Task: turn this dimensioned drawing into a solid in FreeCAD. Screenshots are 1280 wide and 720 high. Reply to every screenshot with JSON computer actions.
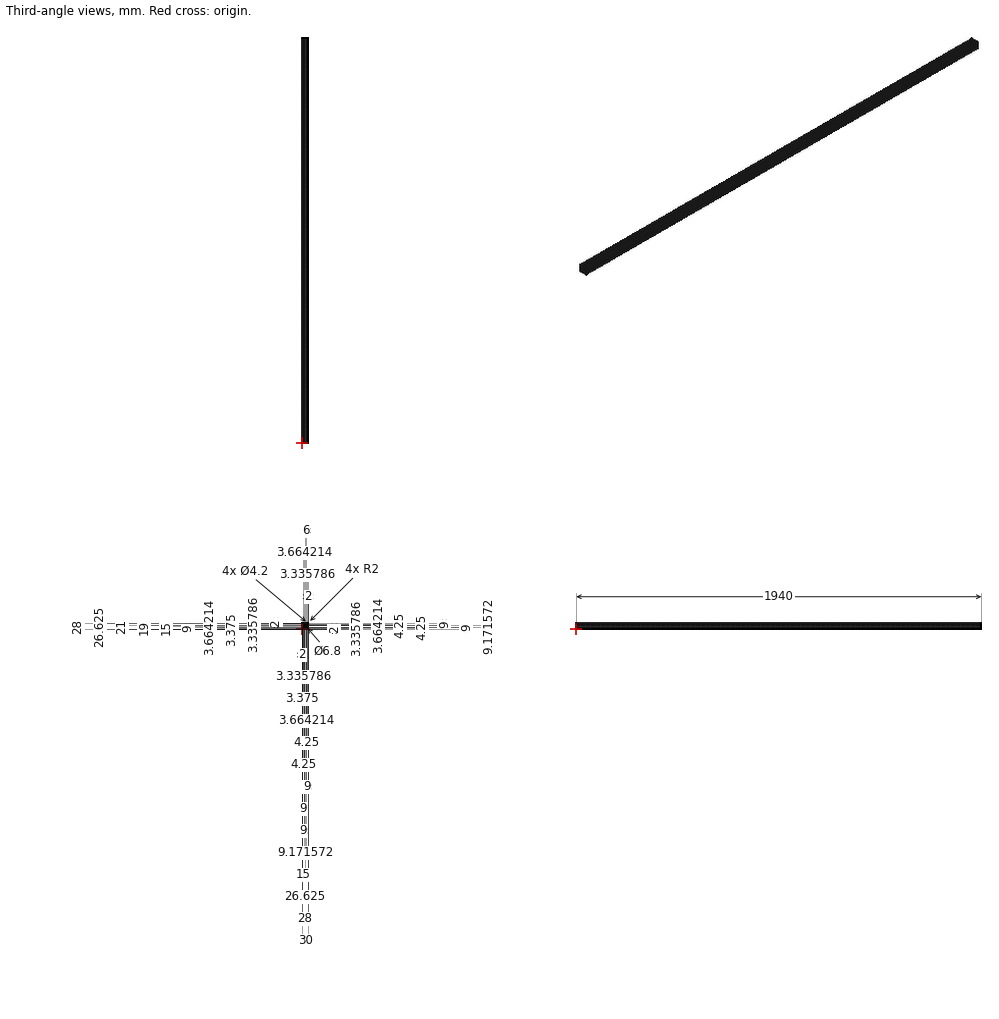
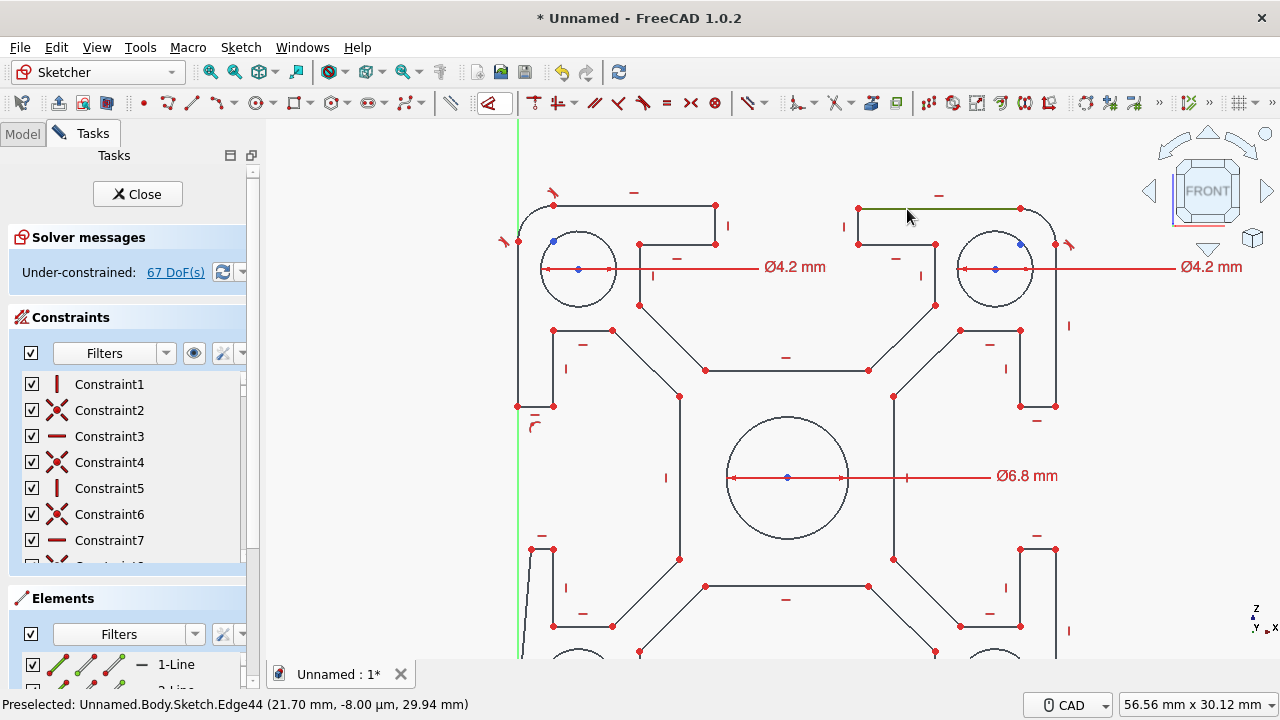
{"action": "left_click", "coordinate": [1052, 228]}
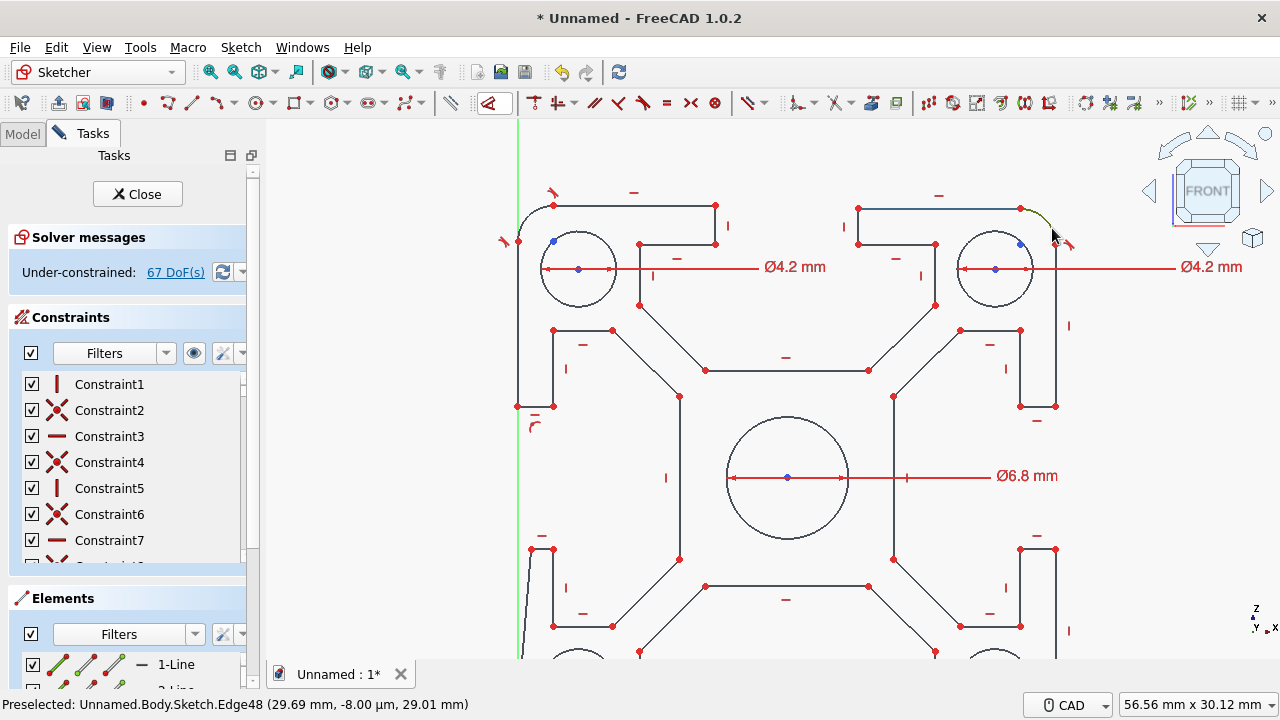
{"action": "left_click", "coordinate": [644, 104]}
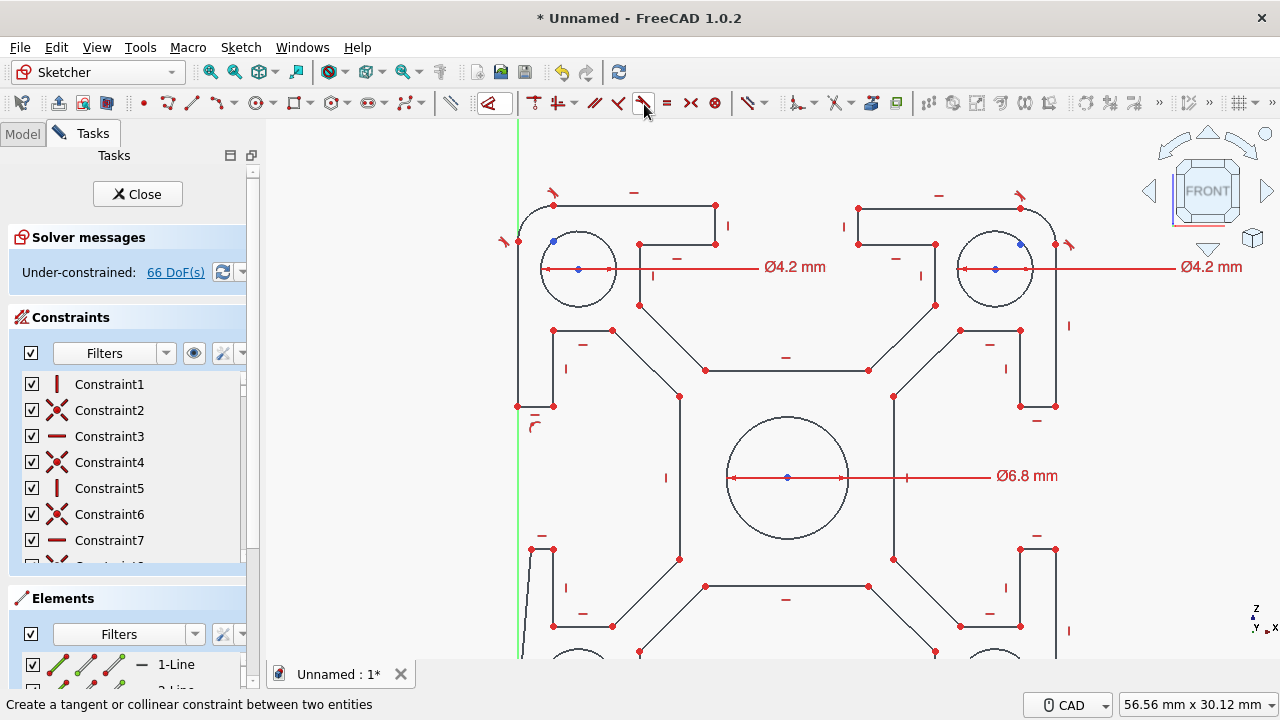
{"action": "scroll", "coordinate": [537, 211], "scroll_direction": "down", "scroll_amount": 2}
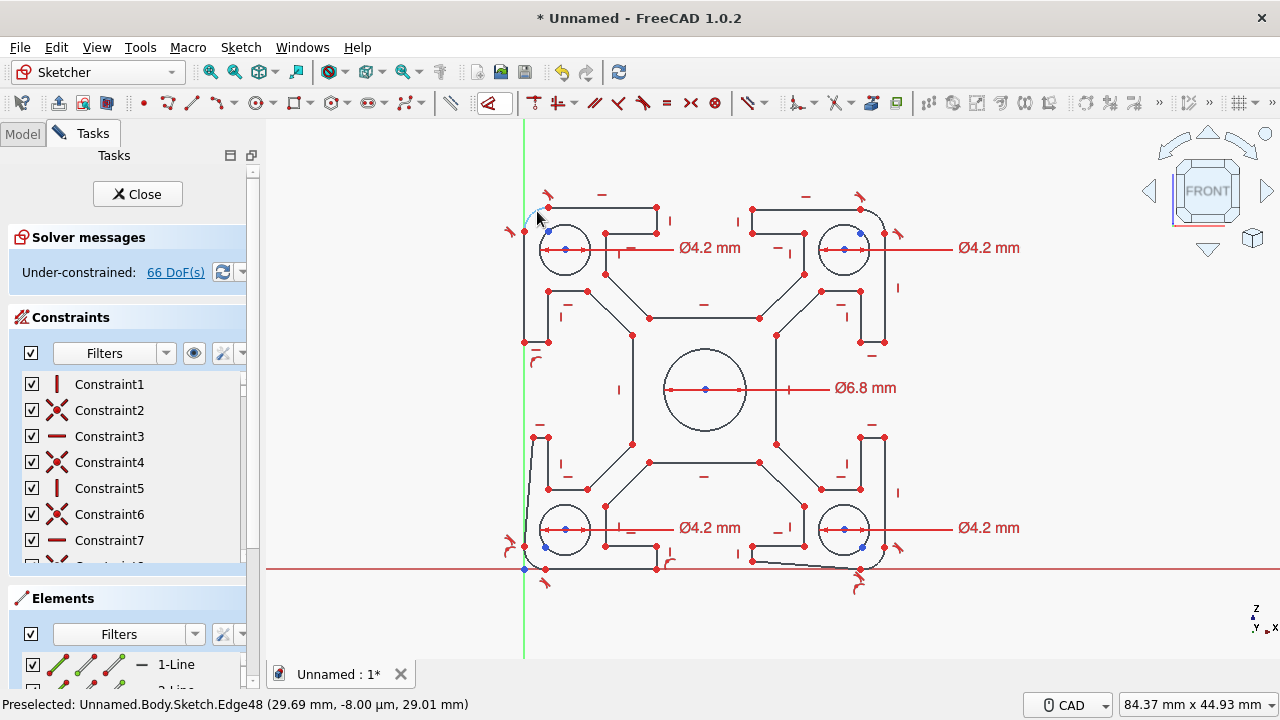
{"action": "left_click", "coordinate": [828, 567]}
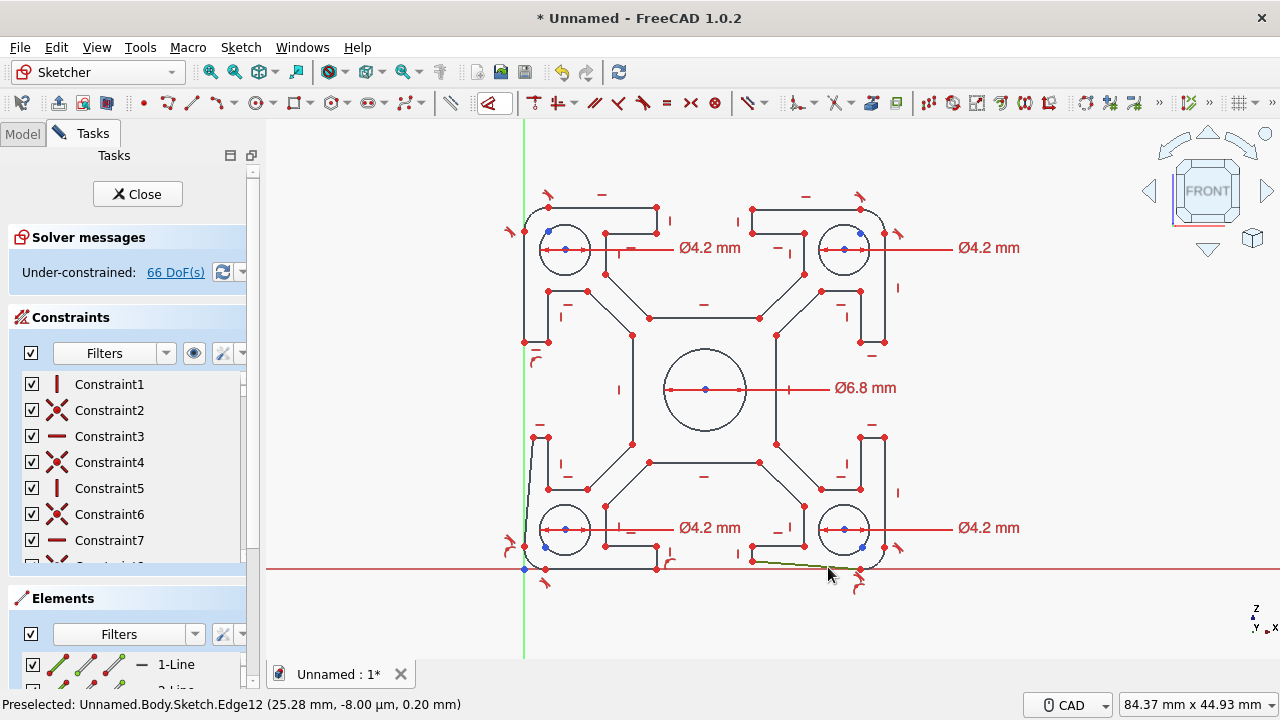
{"action": "left_click", "coordinate": [576, 104]}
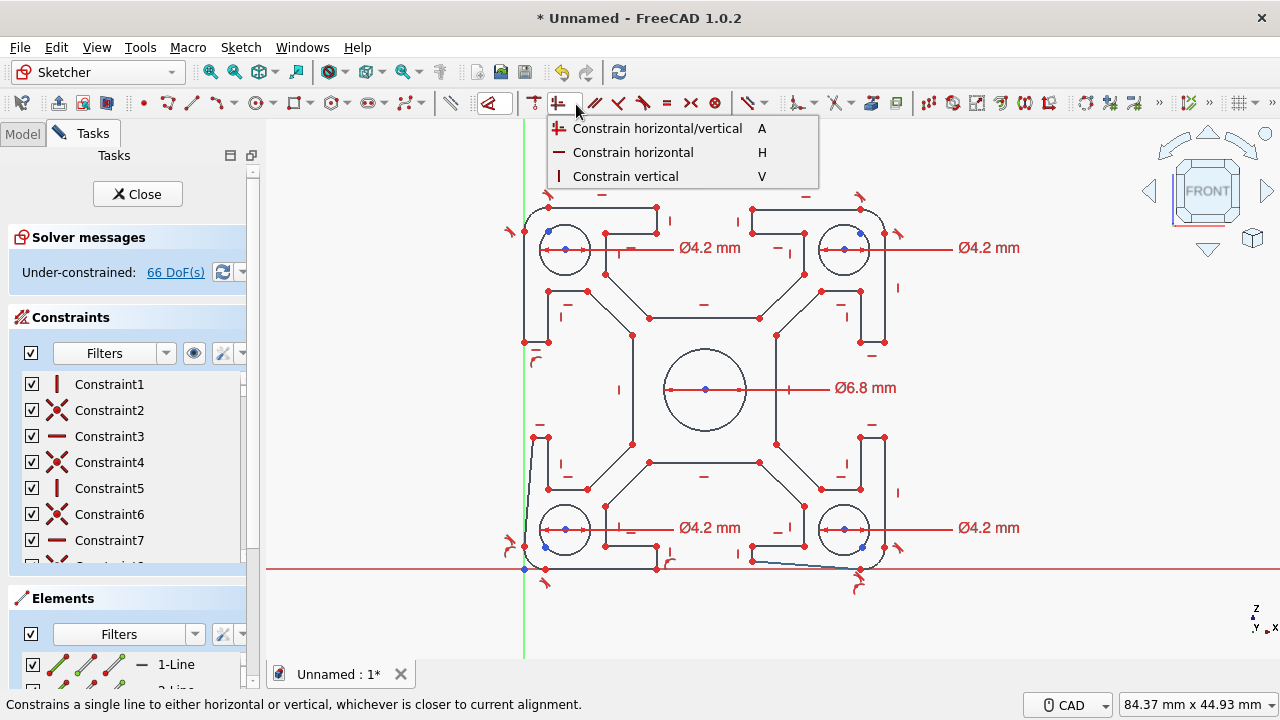
{"action": "left_click", "coordinate": [683, 152]}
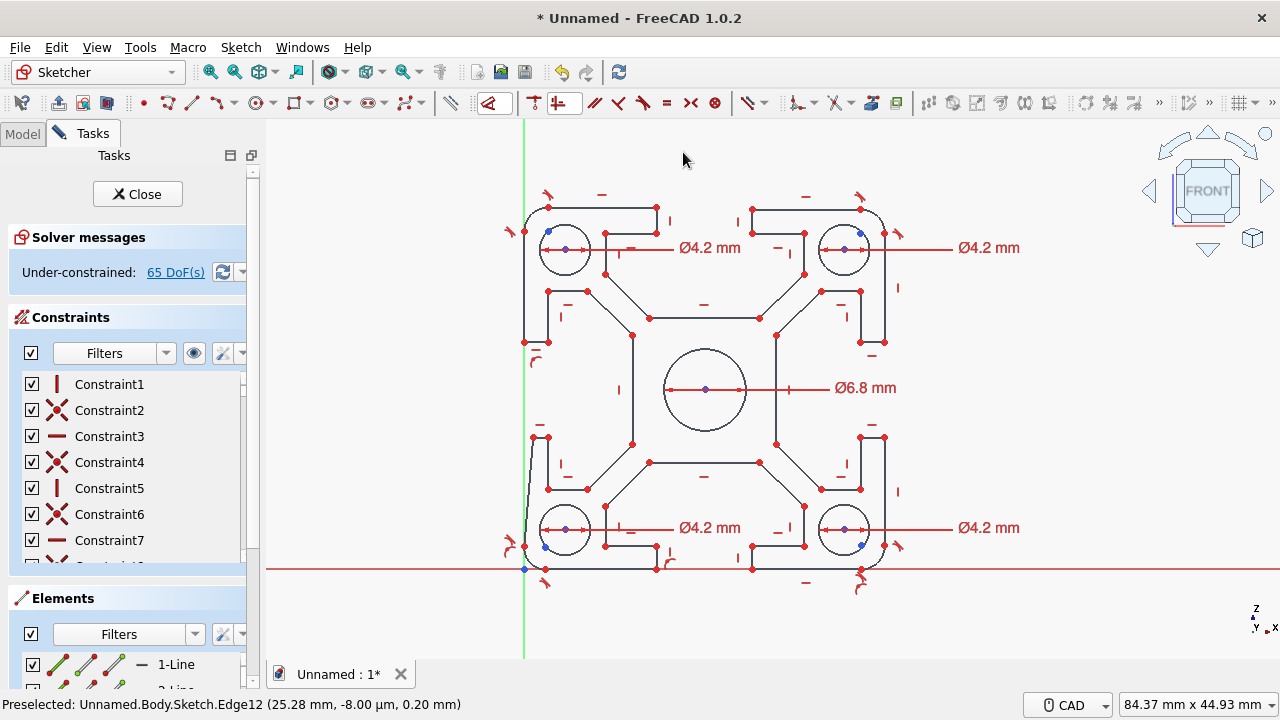
{"action": "left_click", "coordinate": [623, 569]}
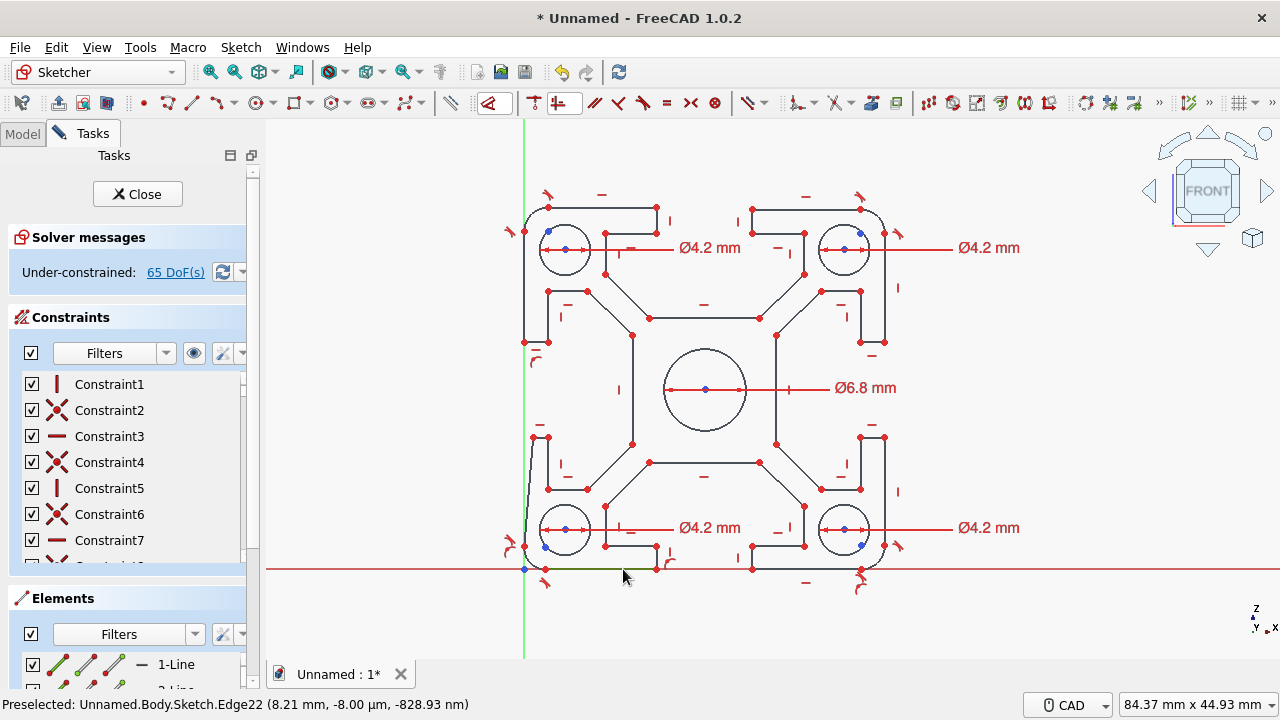
{"action": "key", "text": "h"}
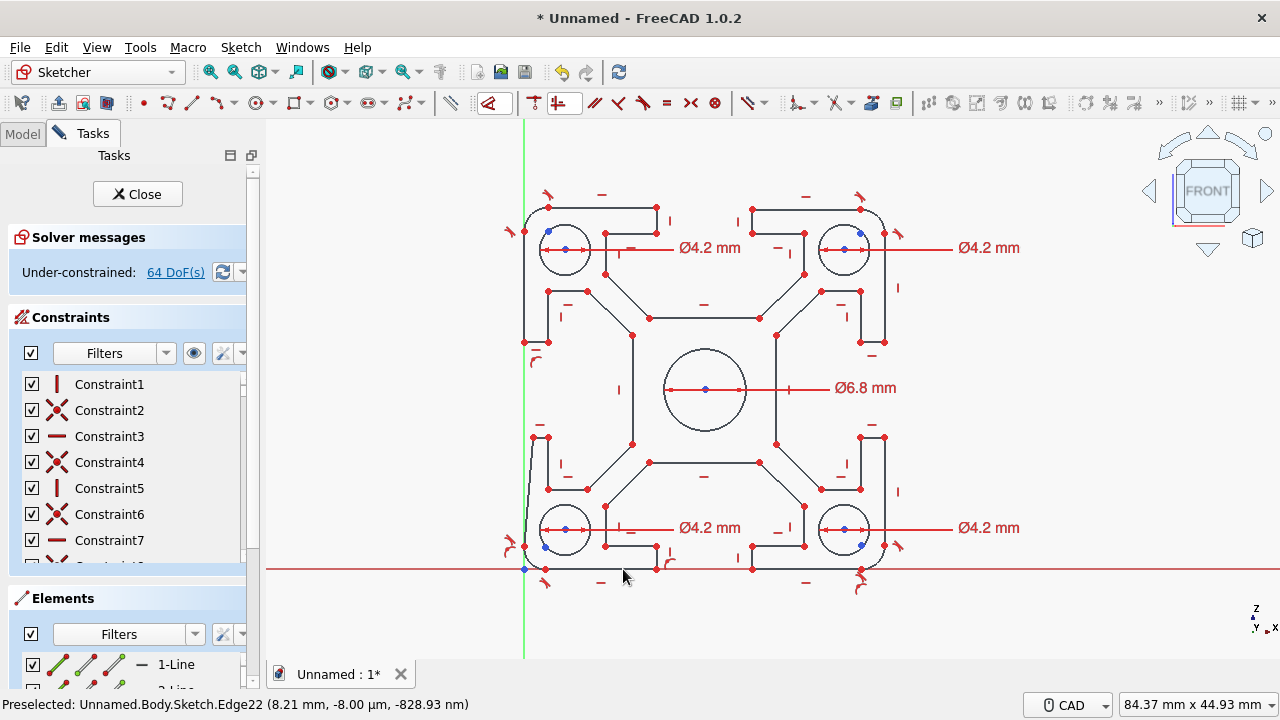
{"action": "left_click", "coordinate": [527, 514]}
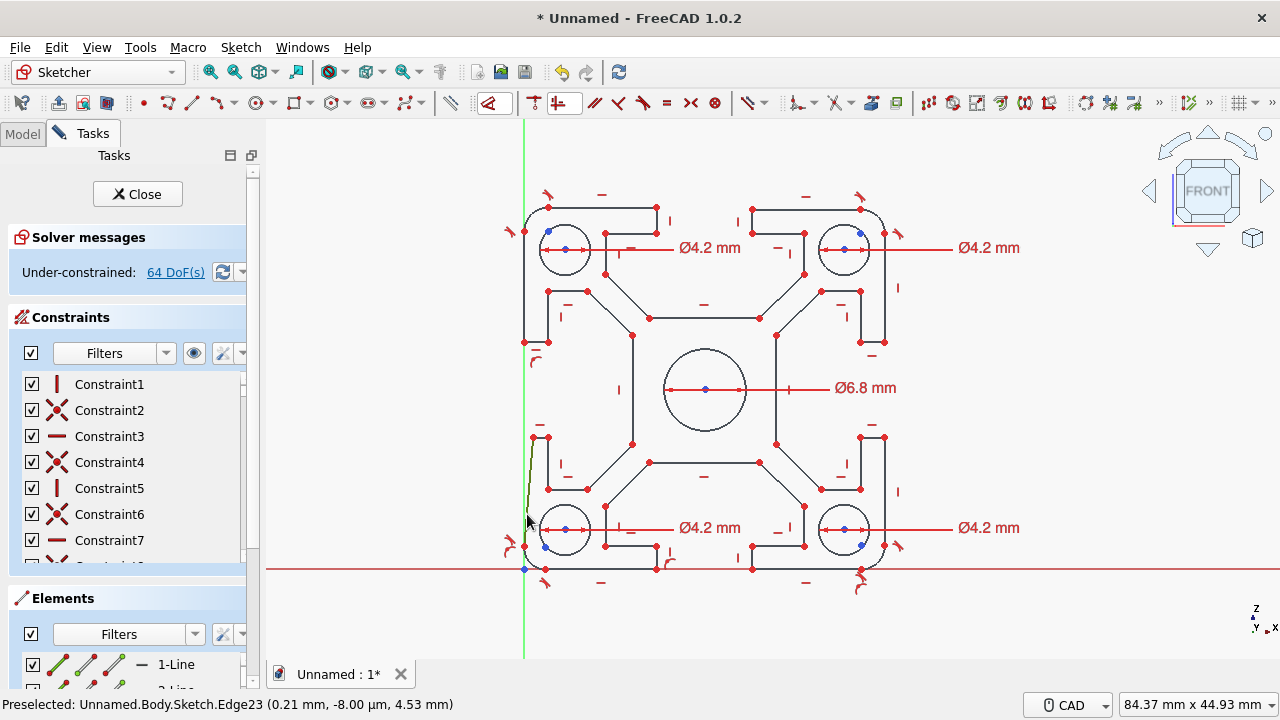
{"action": "key", "text": "v"}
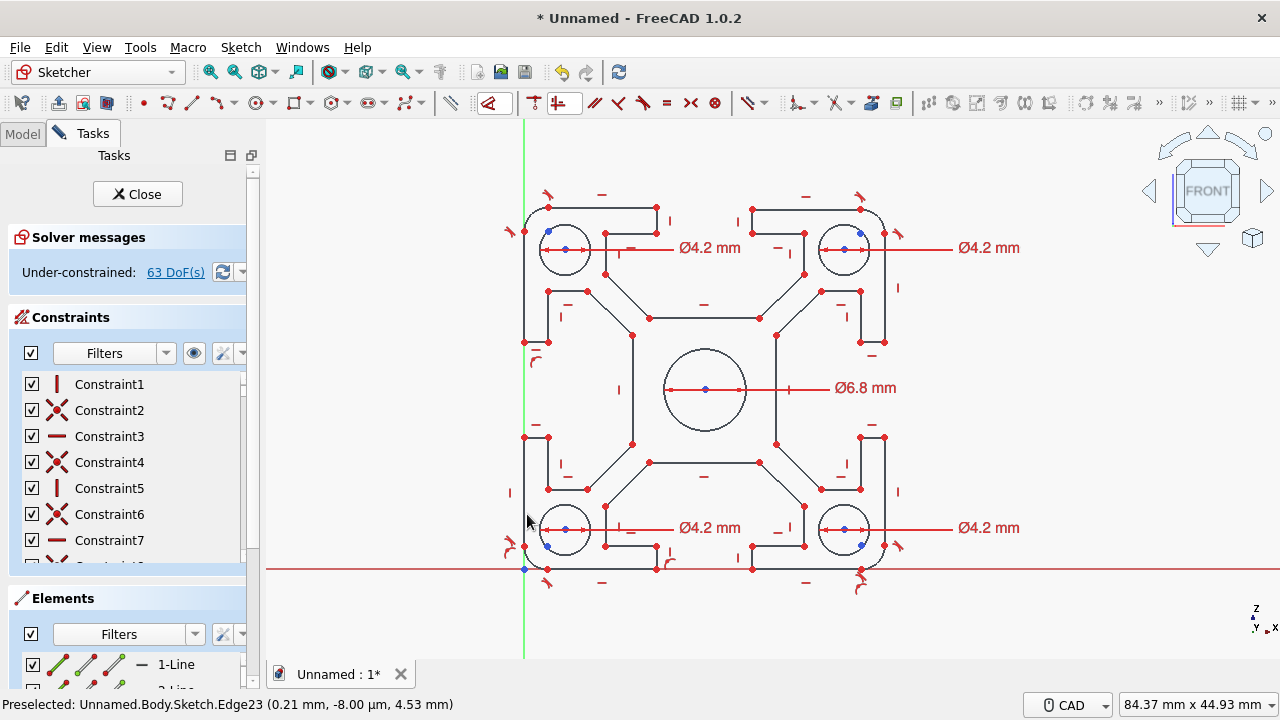
{"action": "left_click", "coordinate": [524, 309]}